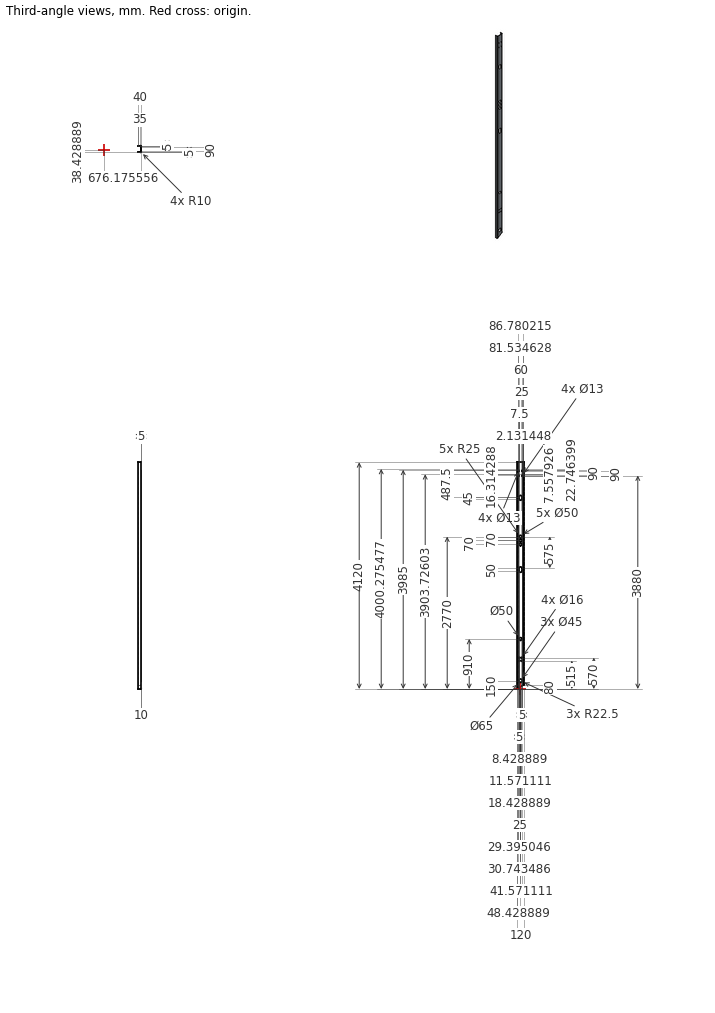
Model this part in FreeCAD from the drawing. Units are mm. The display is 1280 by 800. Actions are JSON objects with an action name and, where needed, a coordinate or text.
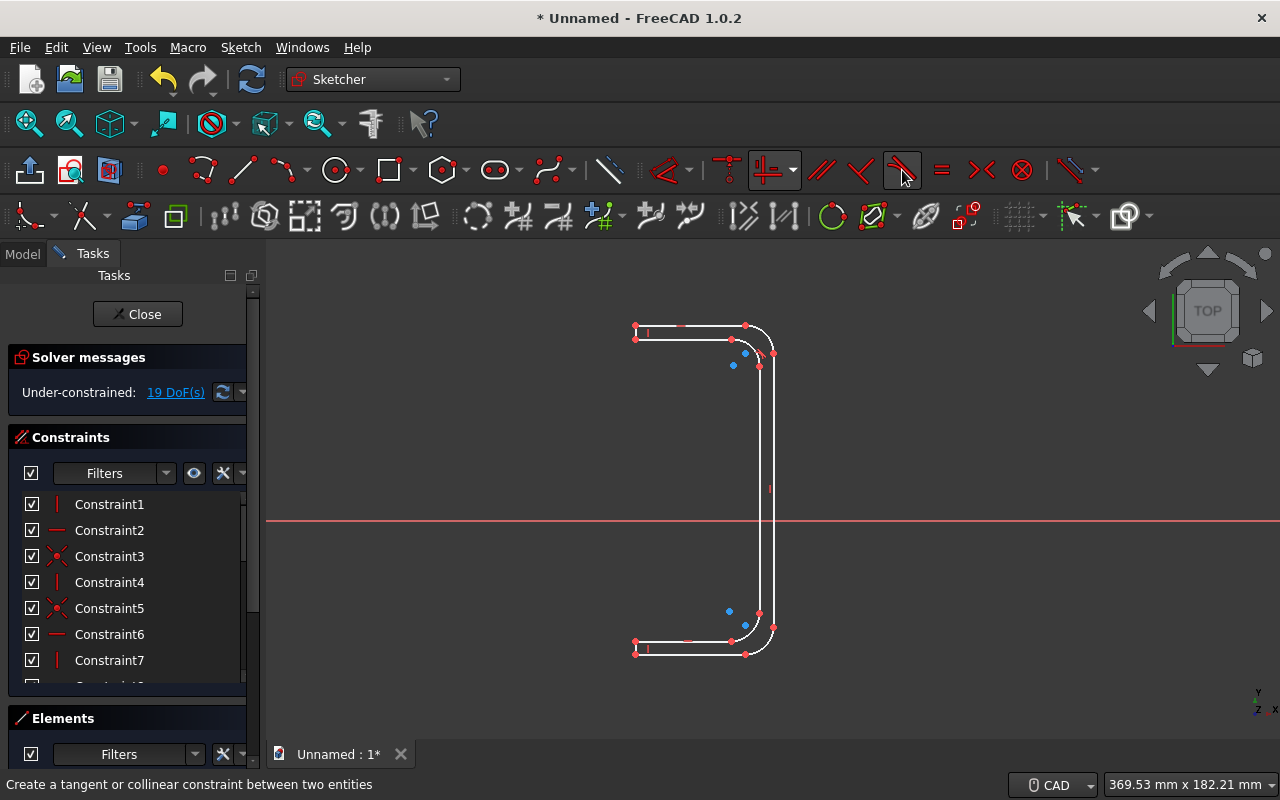
{"action": "left_click", "coordinate": [774, 545]}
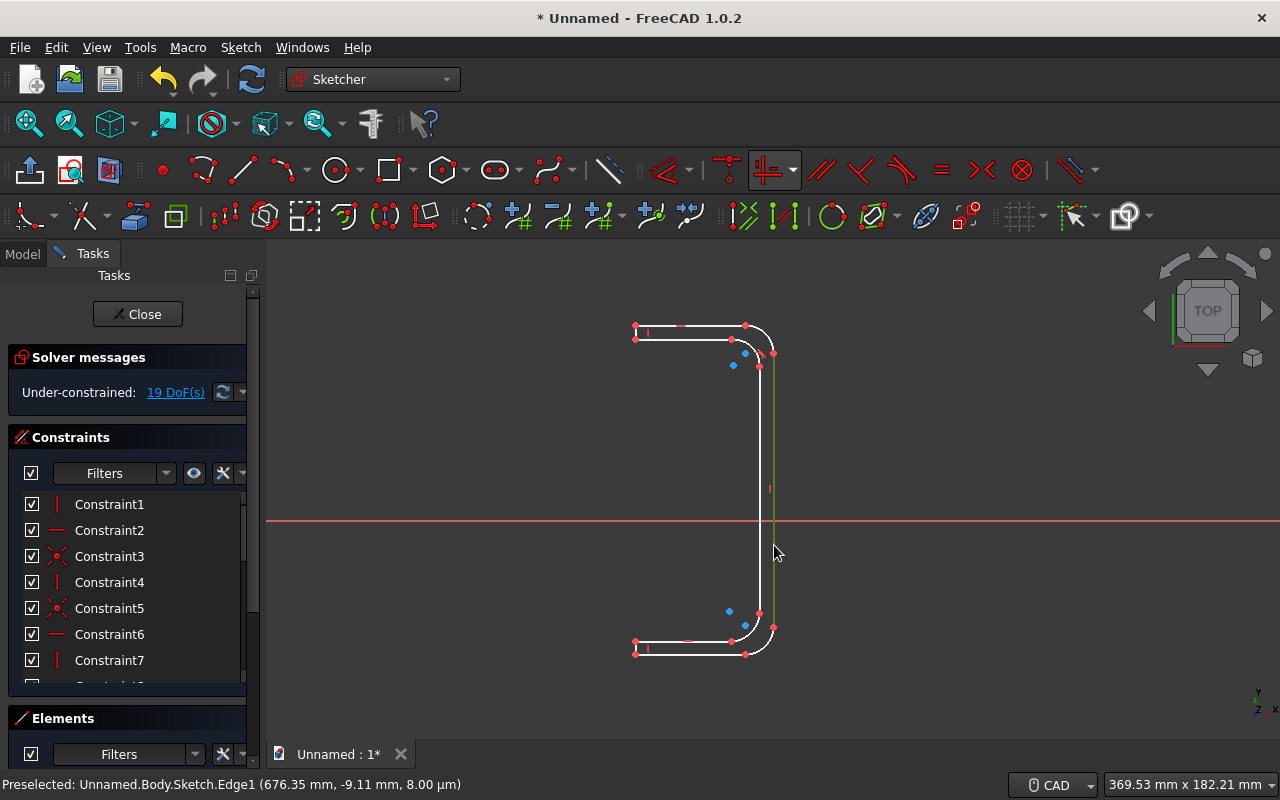
{"action": "left_click", "coordinate": [758, 652]}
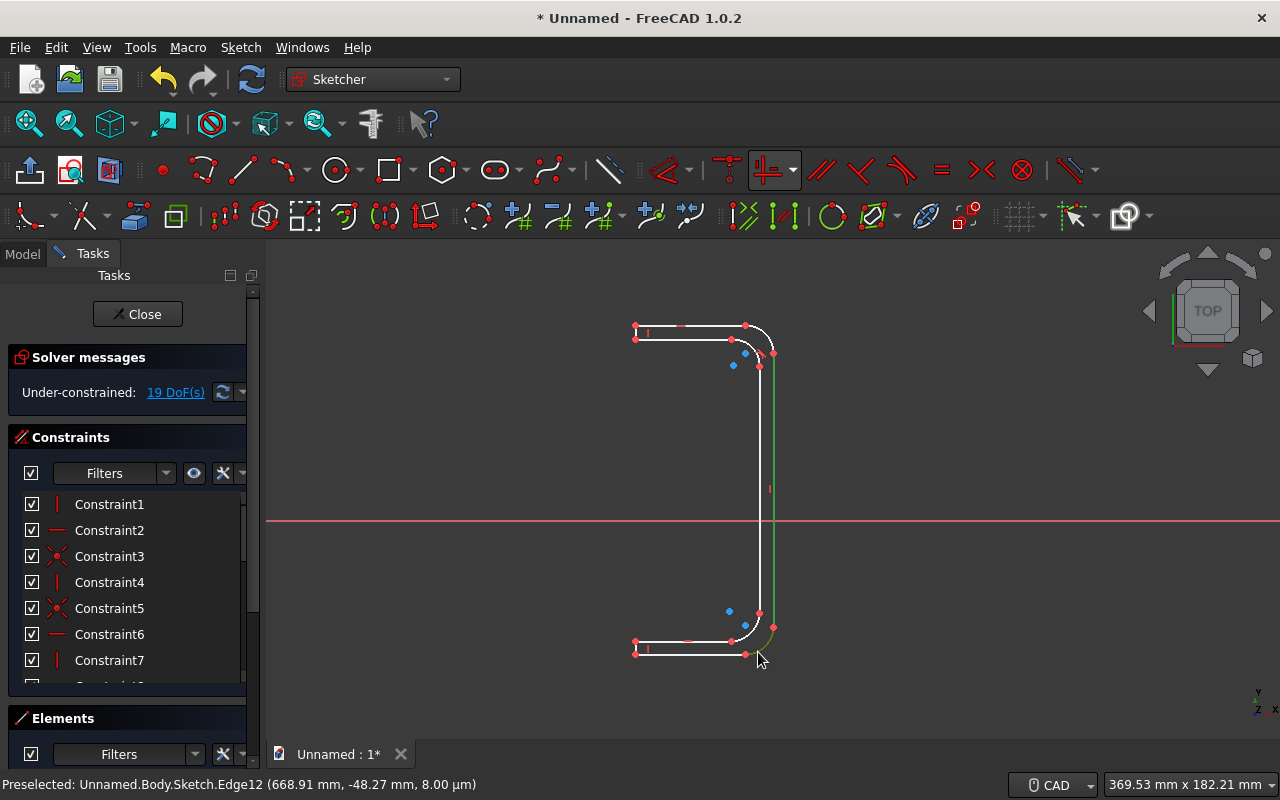
{"action": "key", "text": "t"}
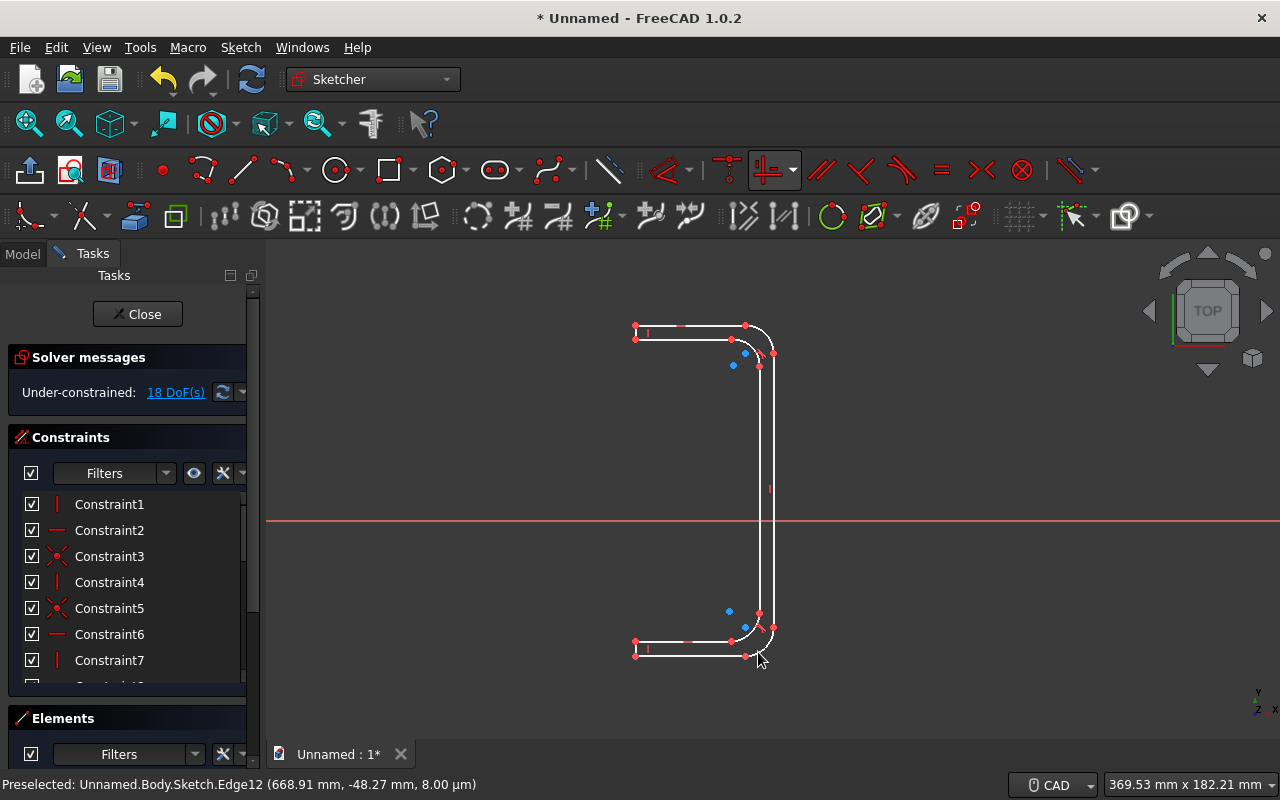
{"action": "left_click", "coordinate": [713, 326]}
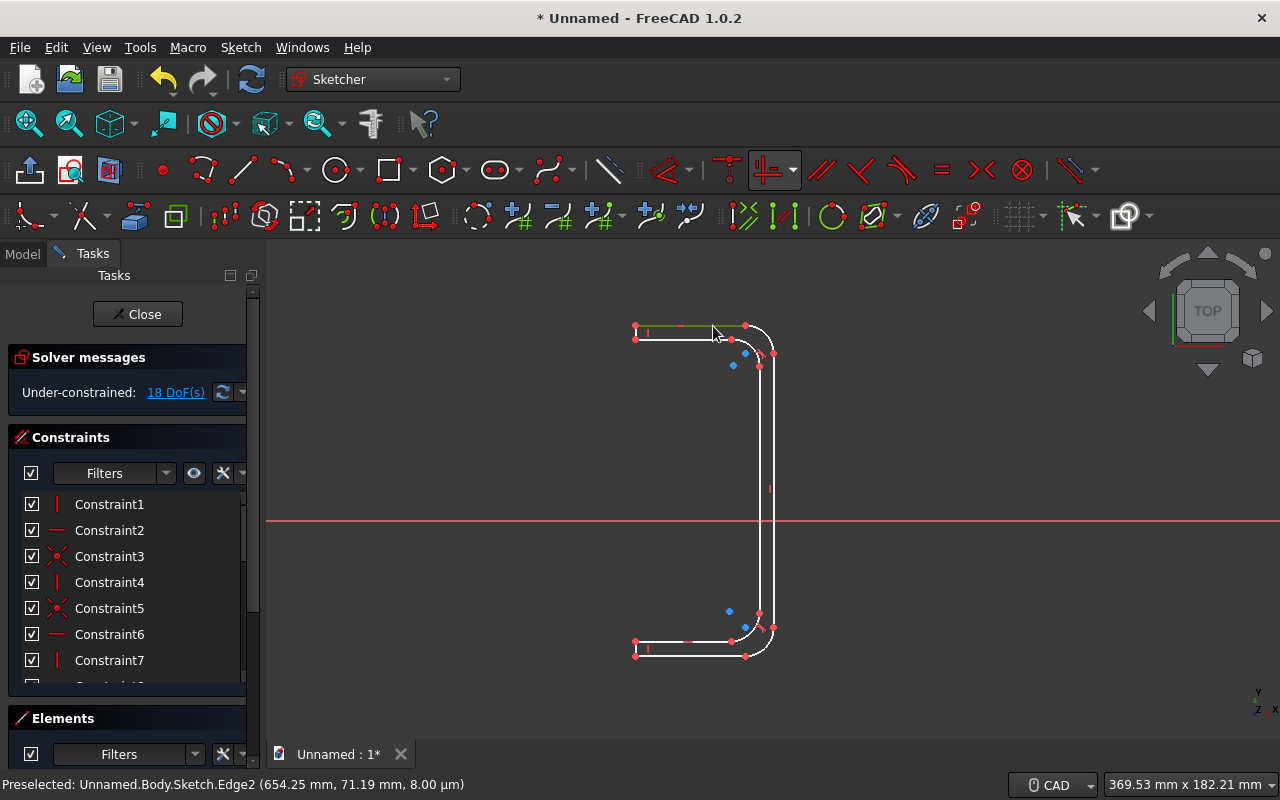
{"action": "left_click", "coordinate": [771, 341]}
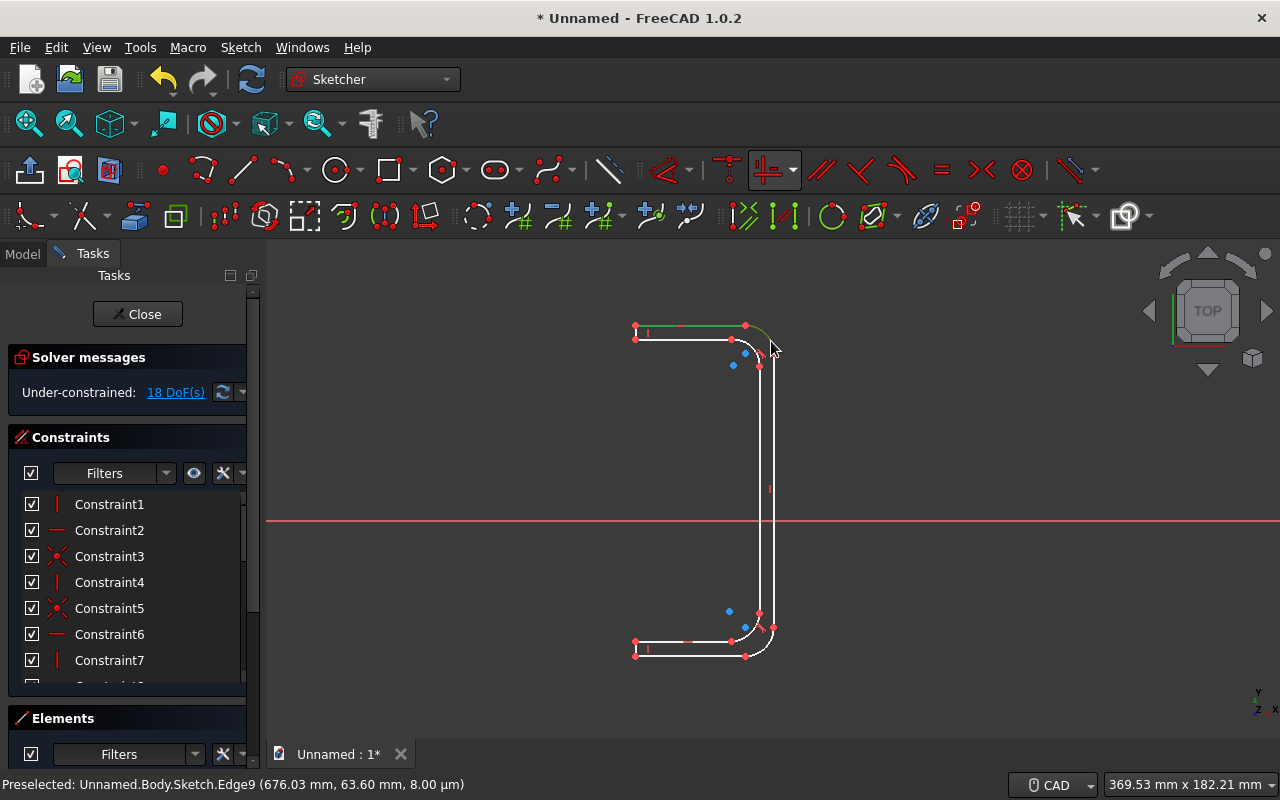
{"action": "key", "text": "t"}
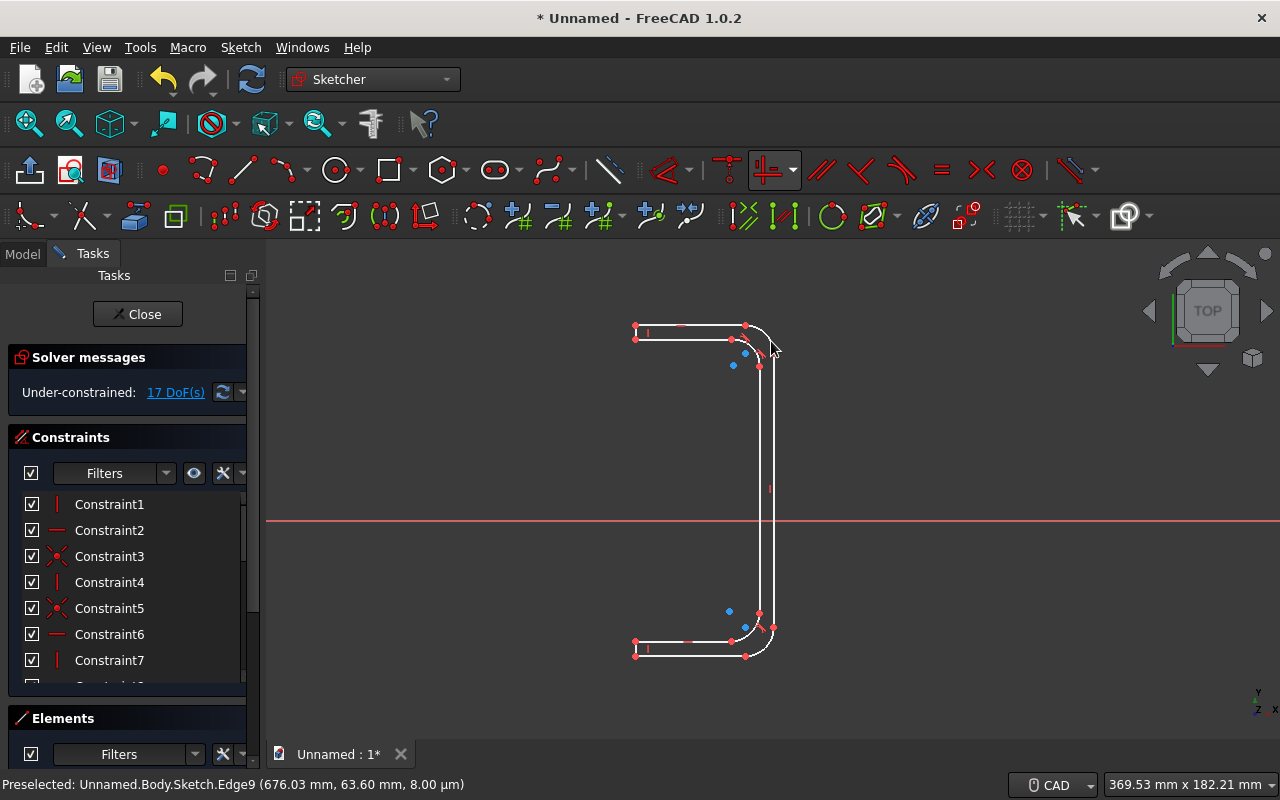
{"action": "left_click", "coordinate": [664, 340]}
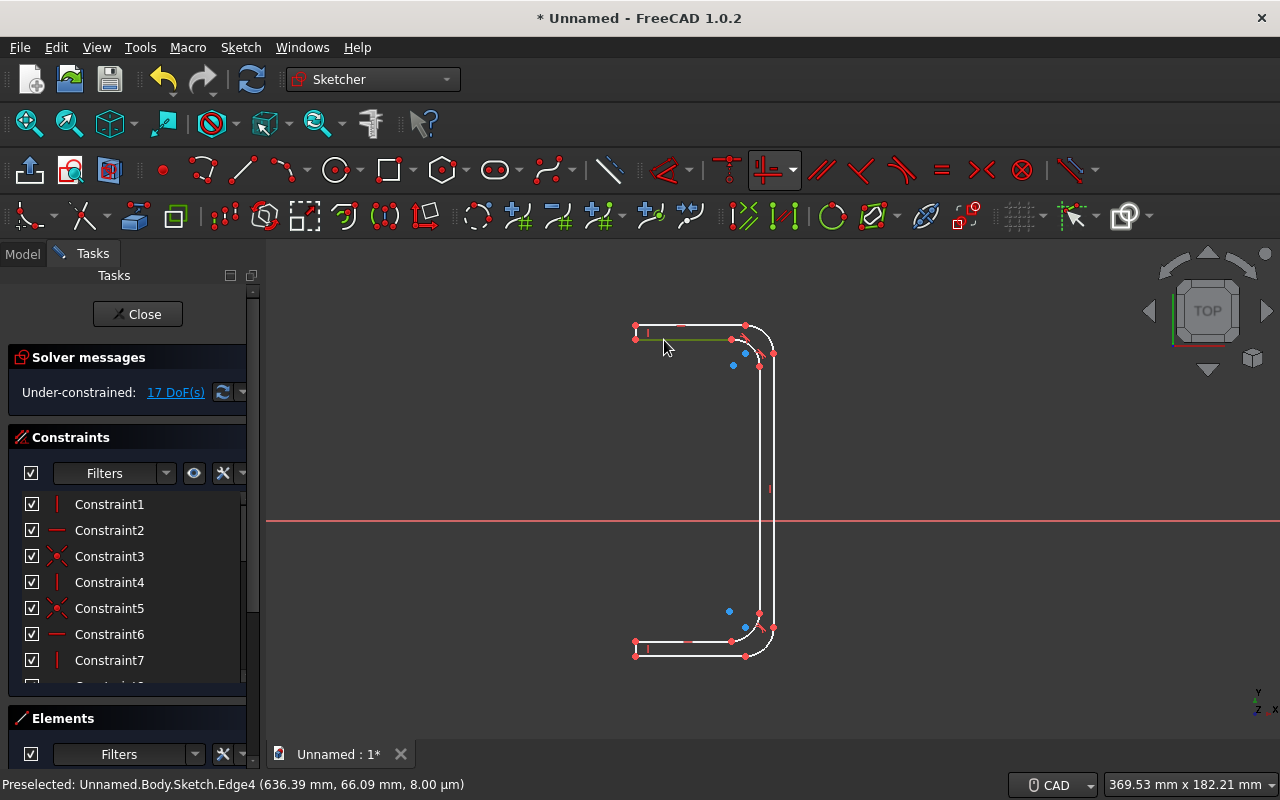
{"action": "left_click", "coordinate": [752, 347]}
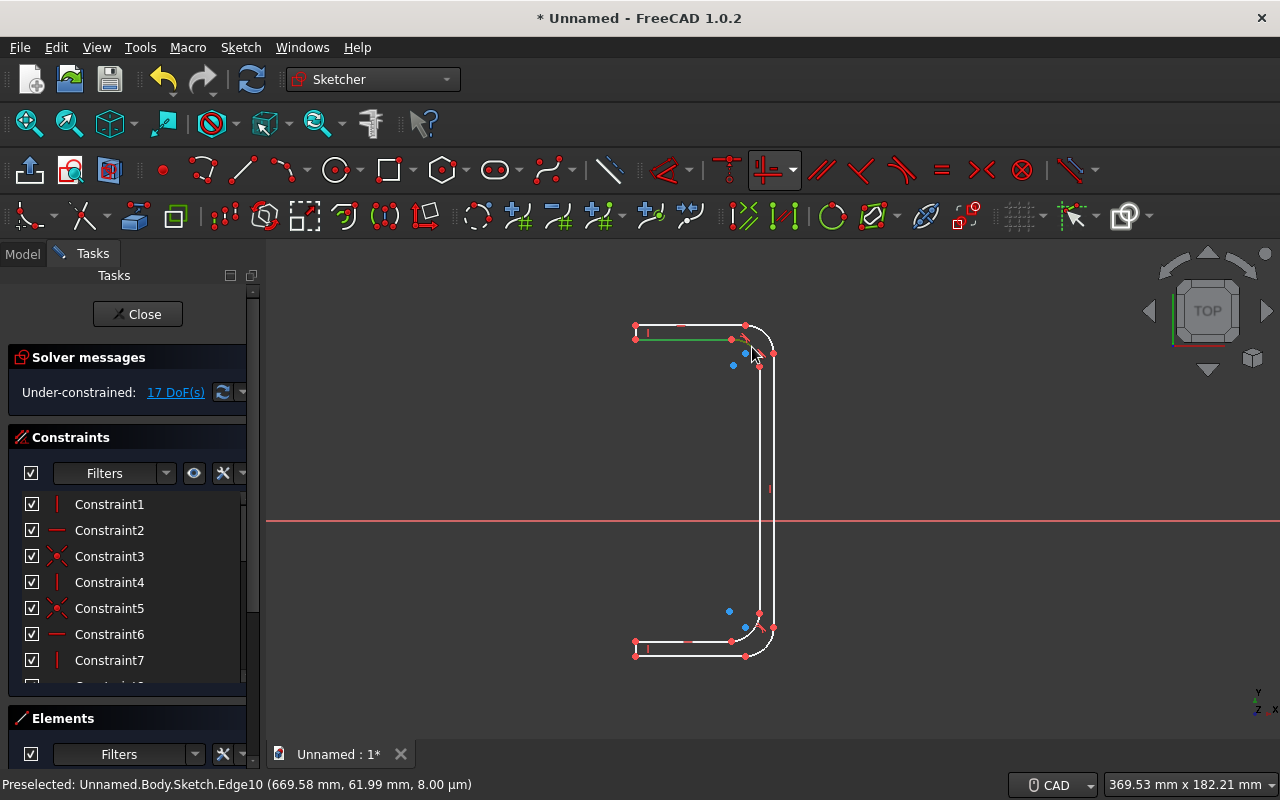
{"action": "left_click", "coordinate": [902, 170]}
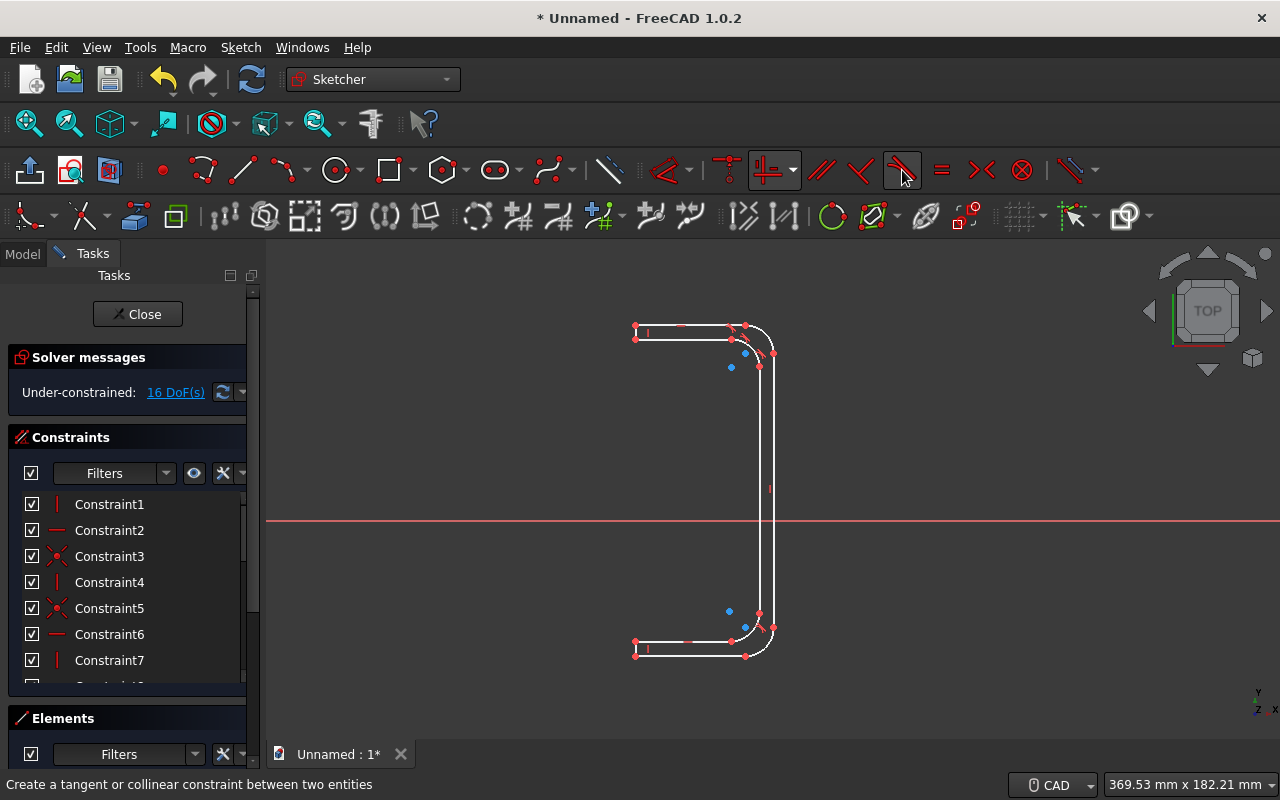
{"action": "left_click", "coordinate": [760, 441]}